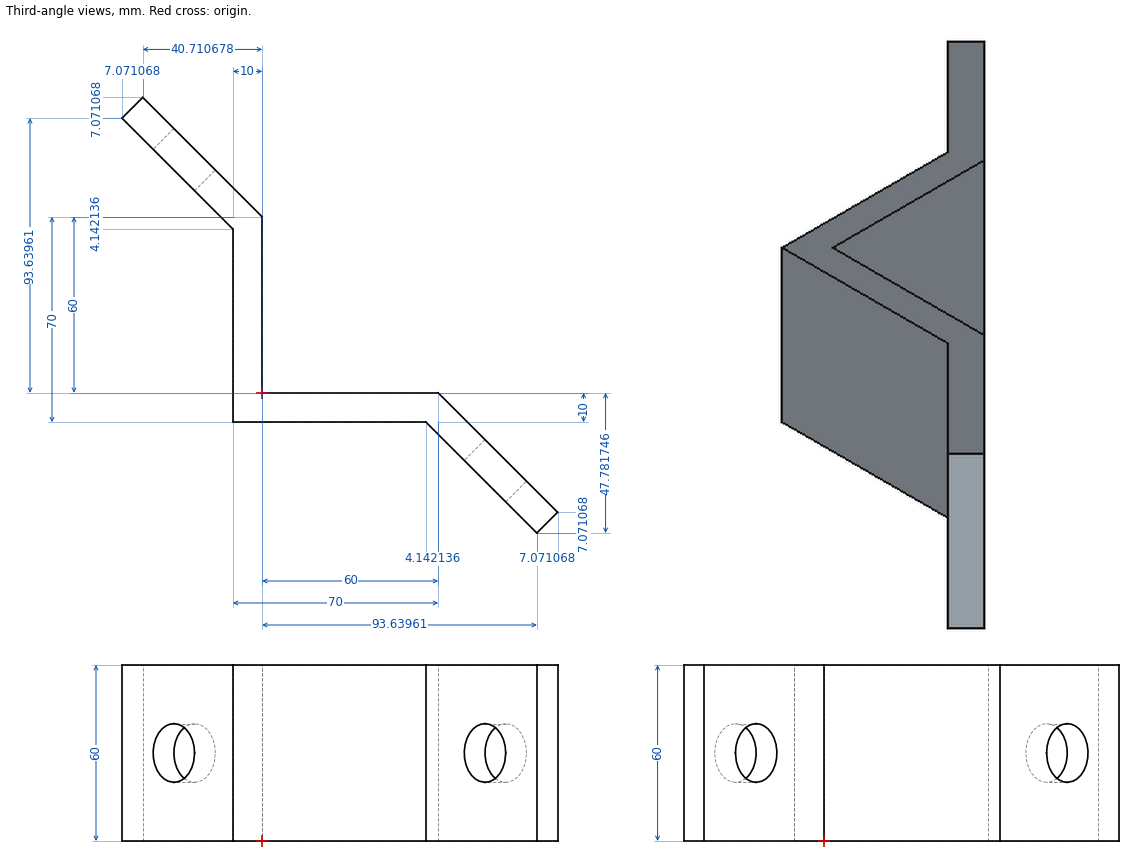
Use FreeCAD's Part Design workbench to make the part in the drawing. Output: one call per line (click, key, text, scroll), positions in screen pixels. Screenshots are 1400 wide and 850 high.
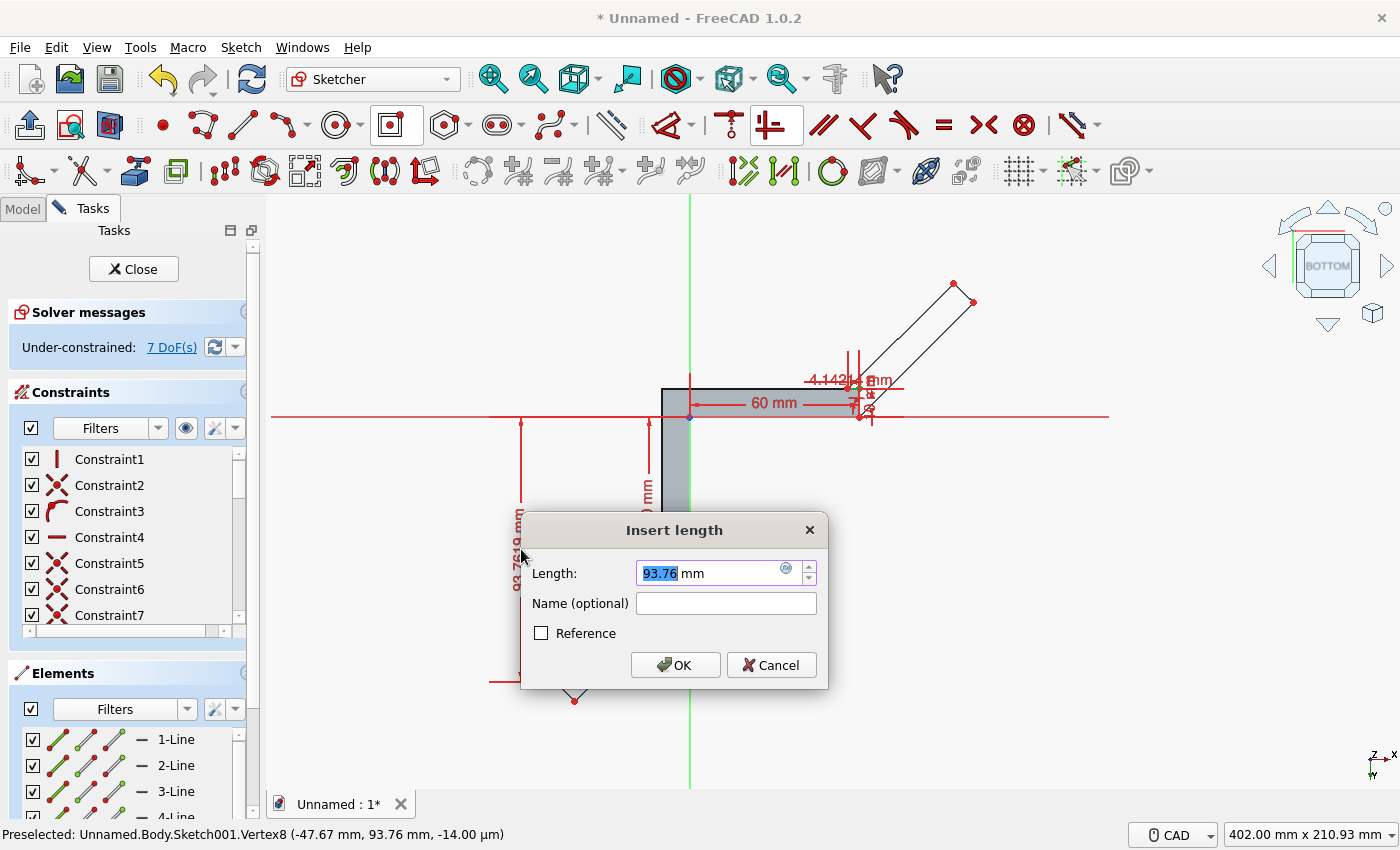
text(93.63961)
key(Return)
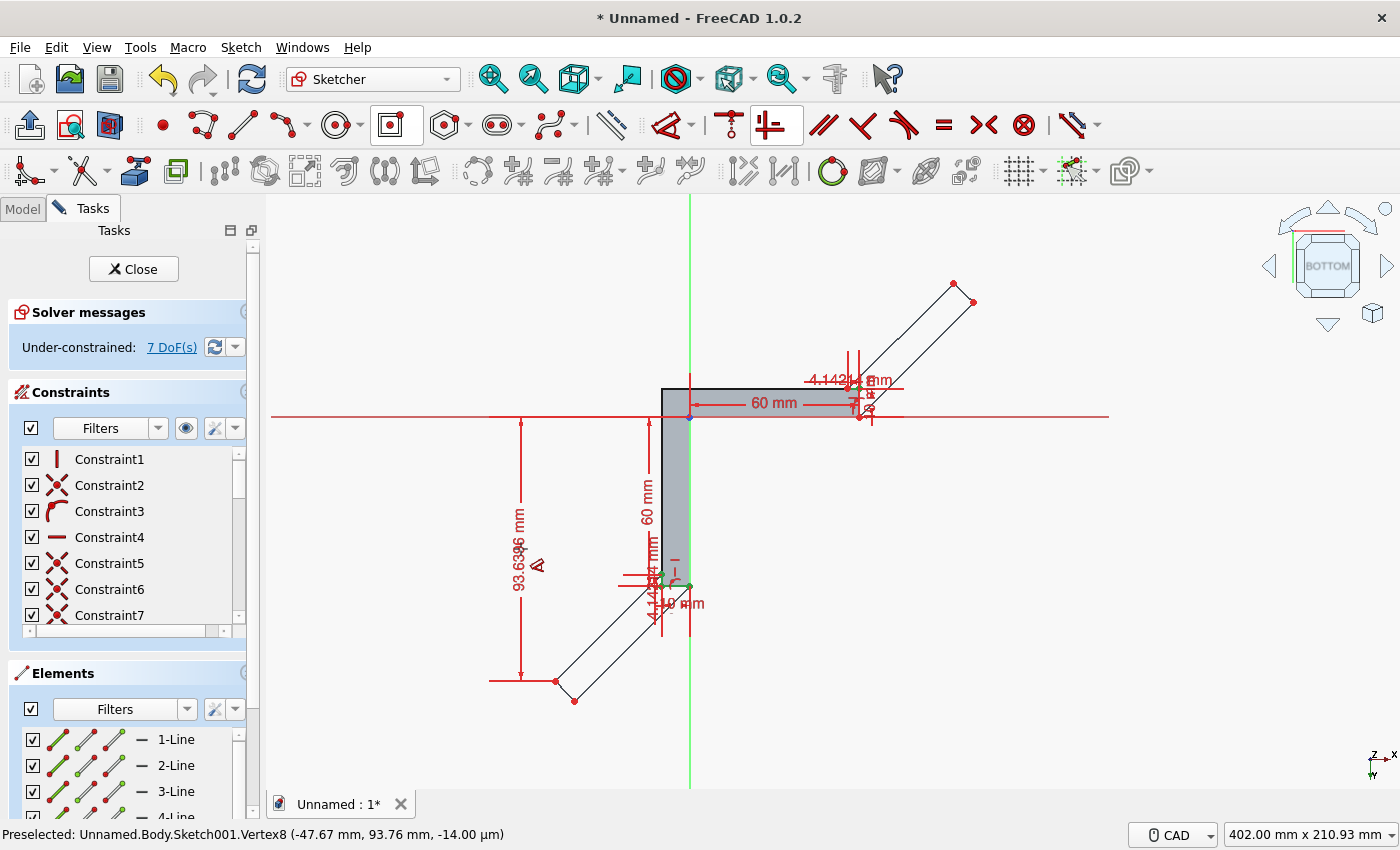
click(954, 284)
click(822, 250)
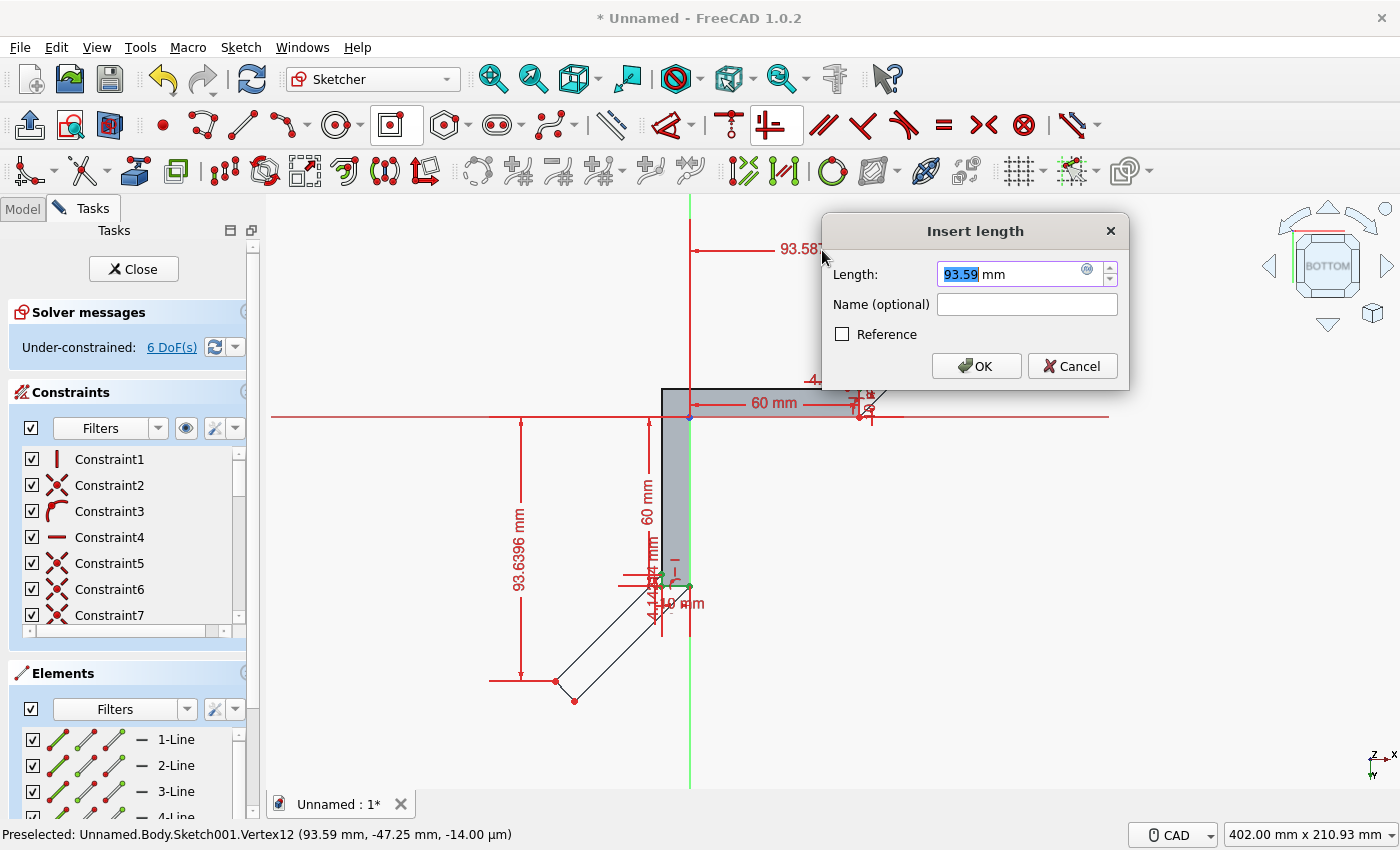
text(93.63961)
key(Return)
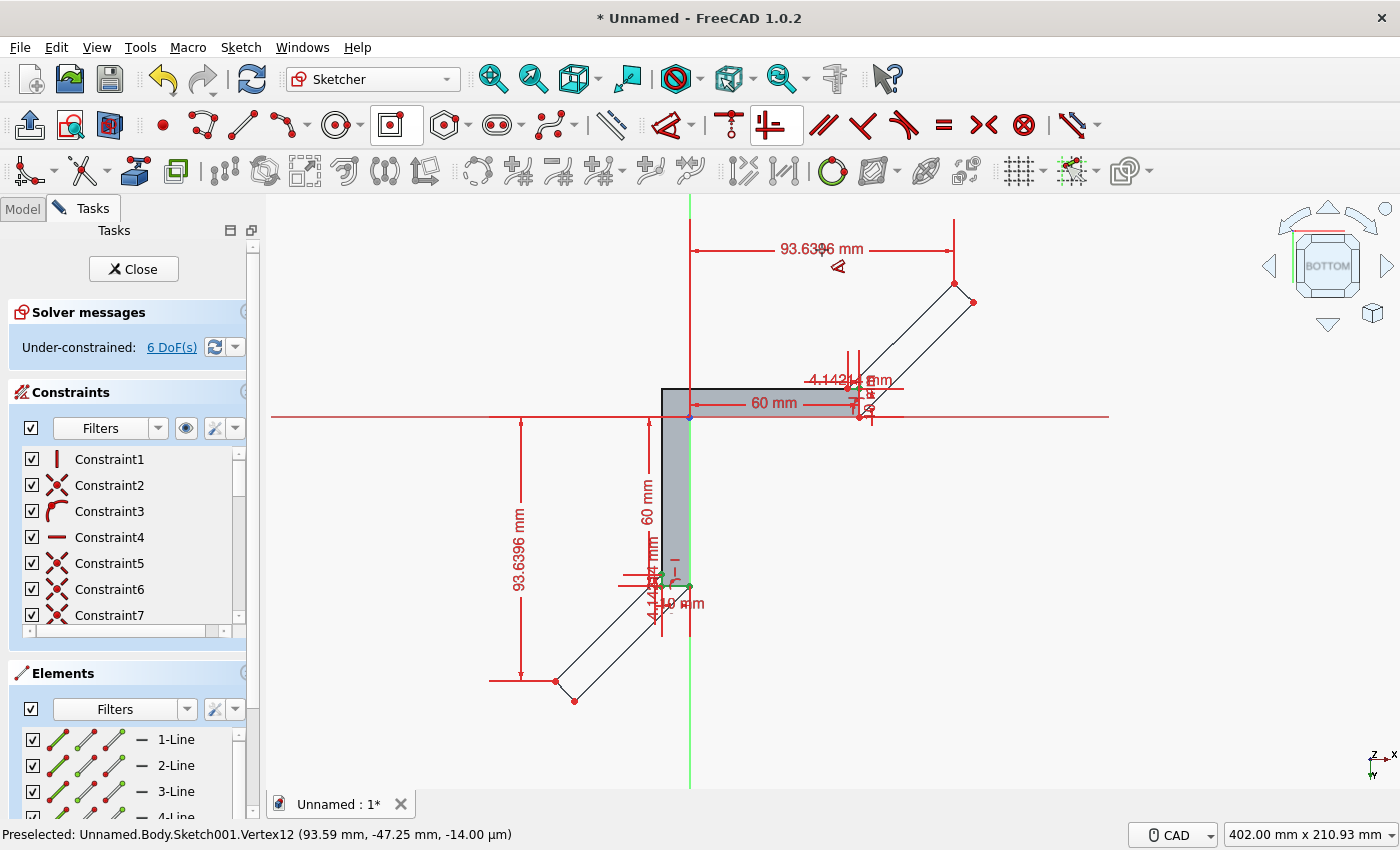
scroll(567, 693, up, 4)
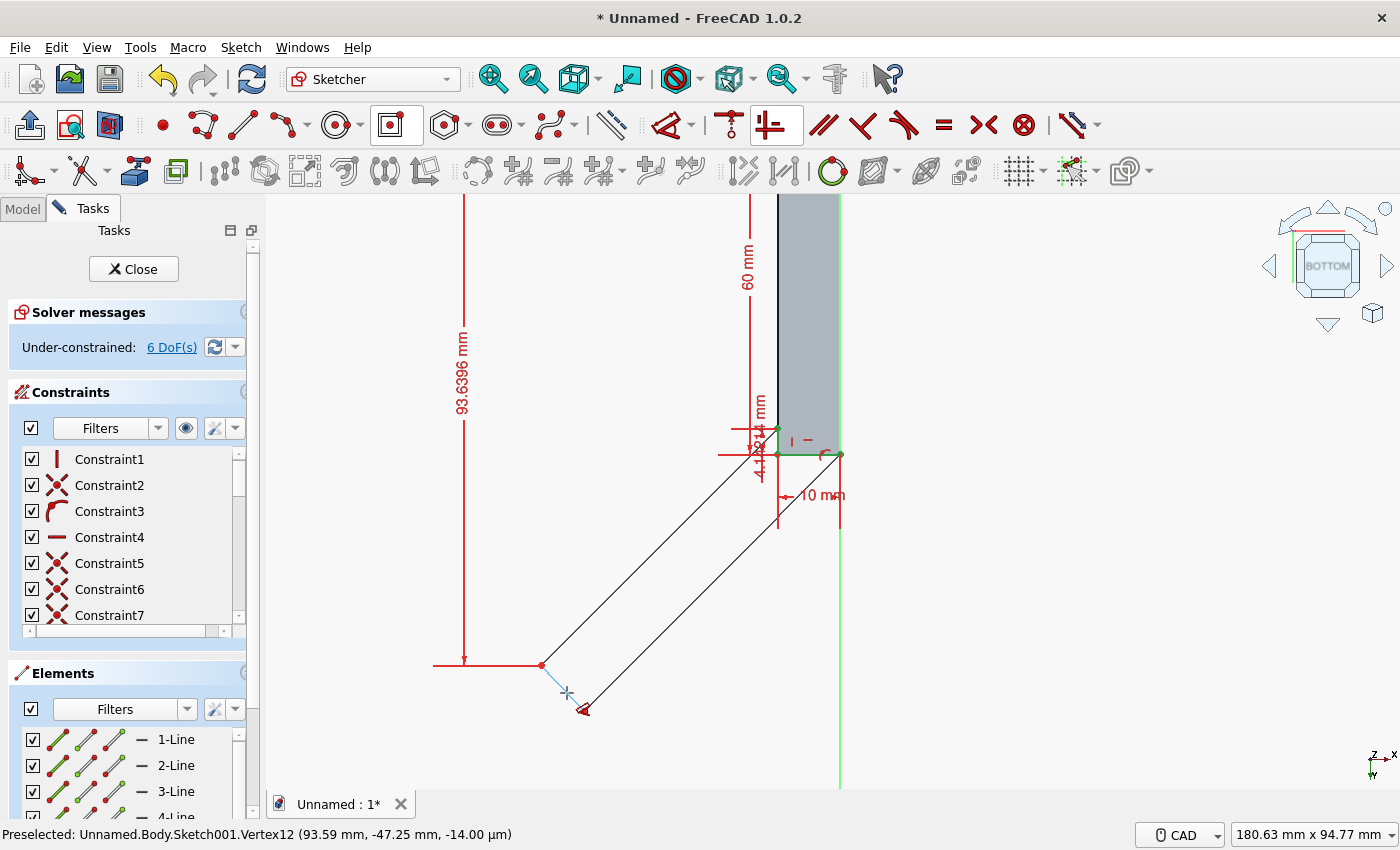
click(567, 693)
click(563, 745)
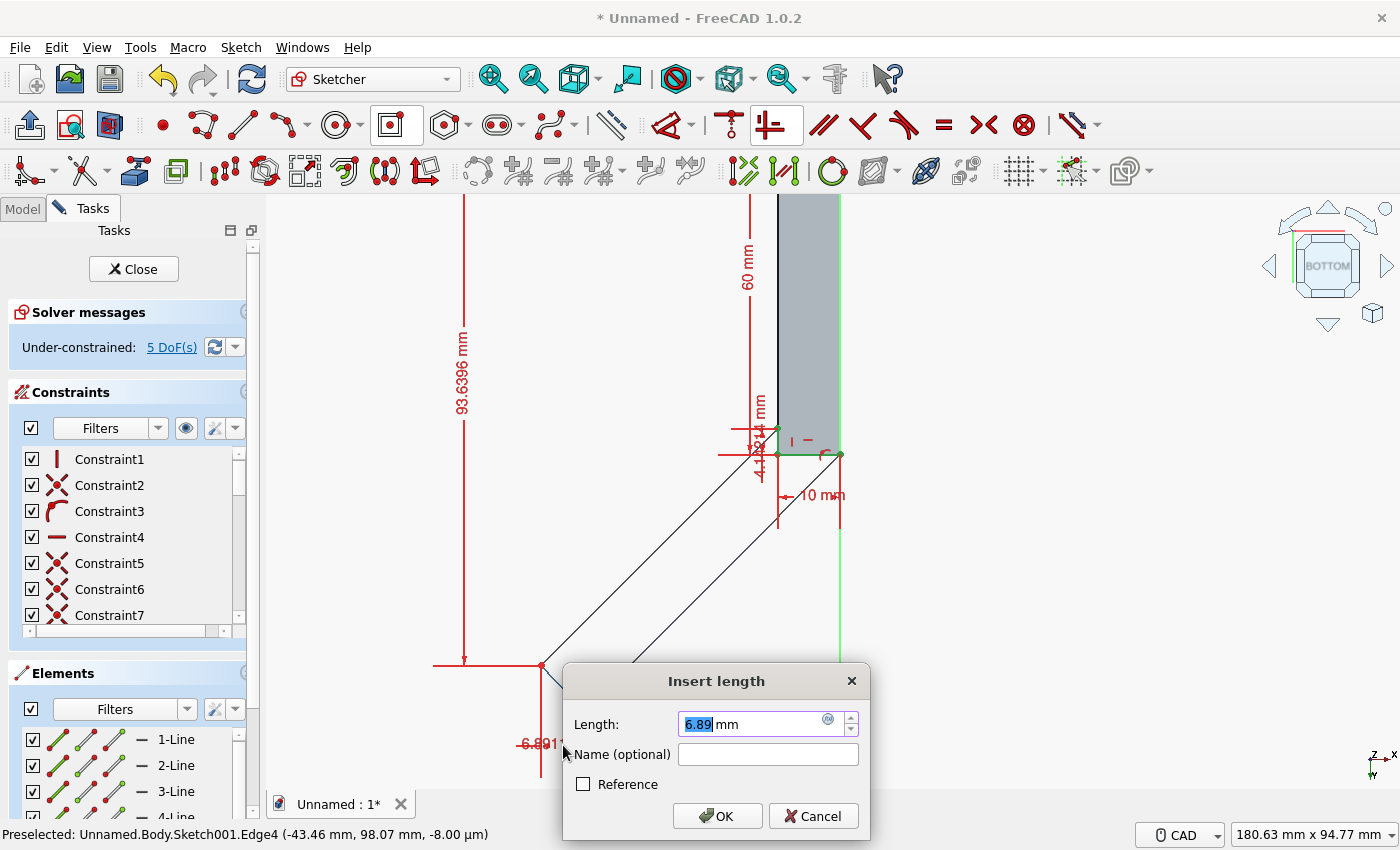
text(7.071068)
key(Return)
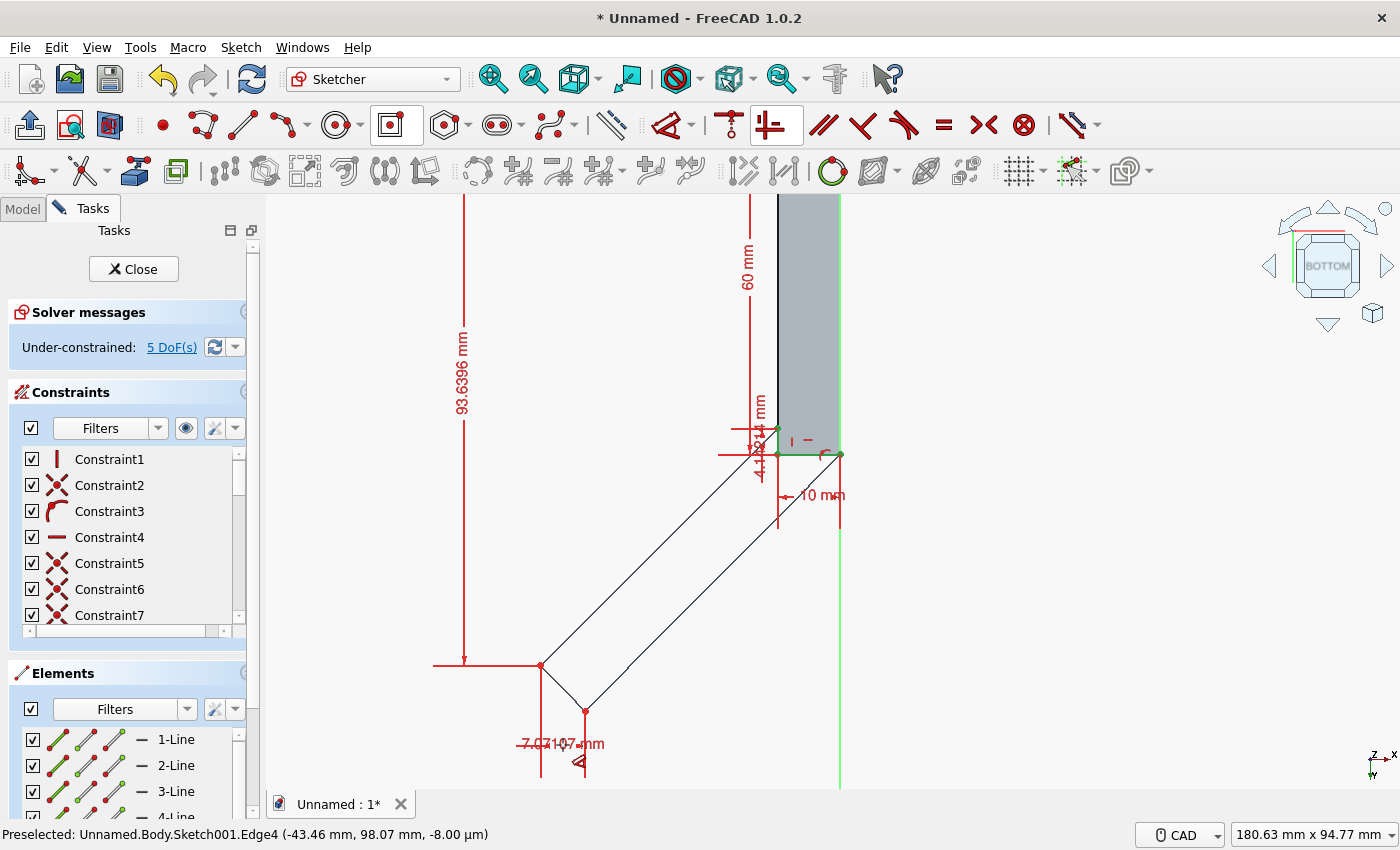
click(572, 698)
click(507, 688)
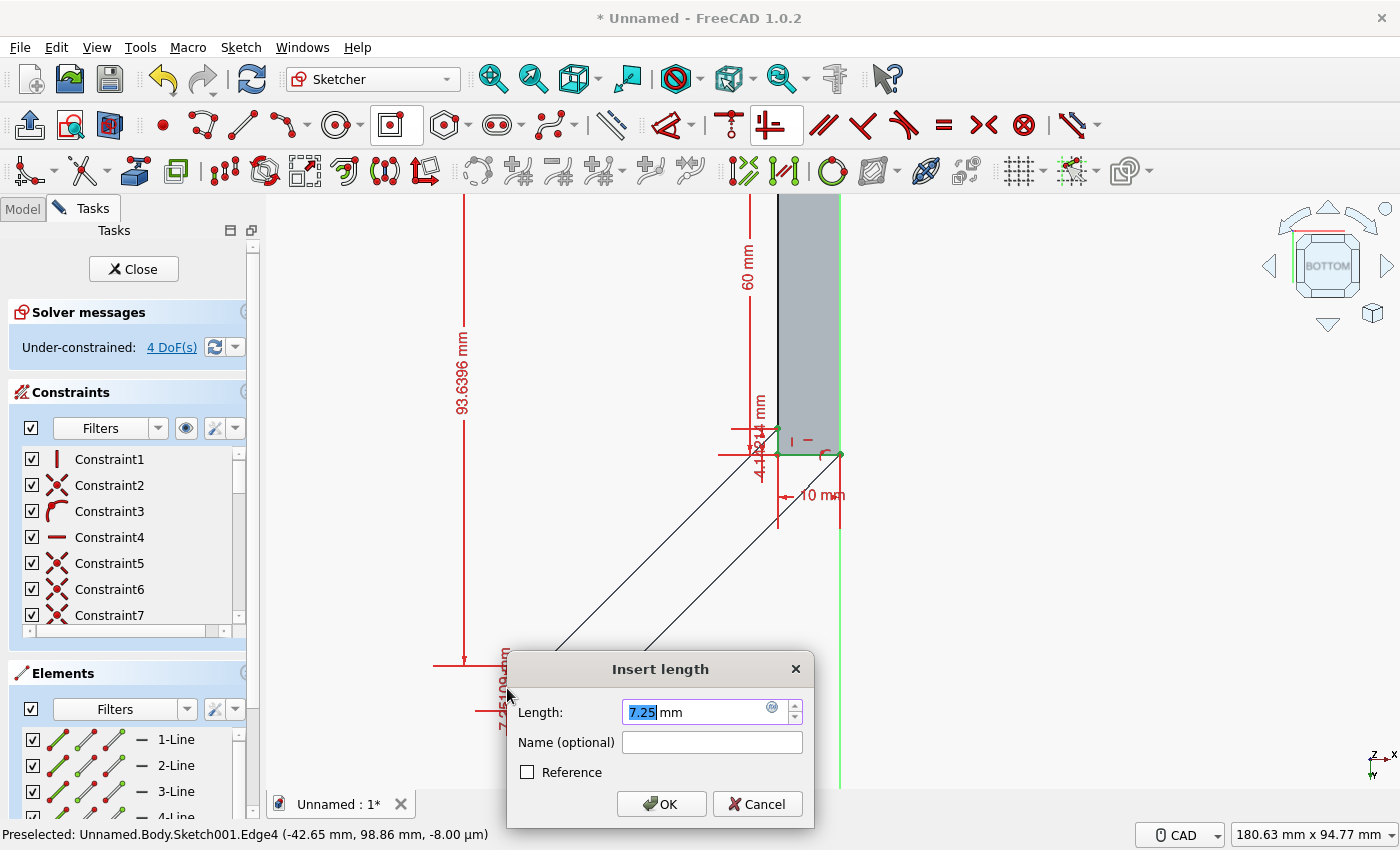
text(7.071068)
key(Return)